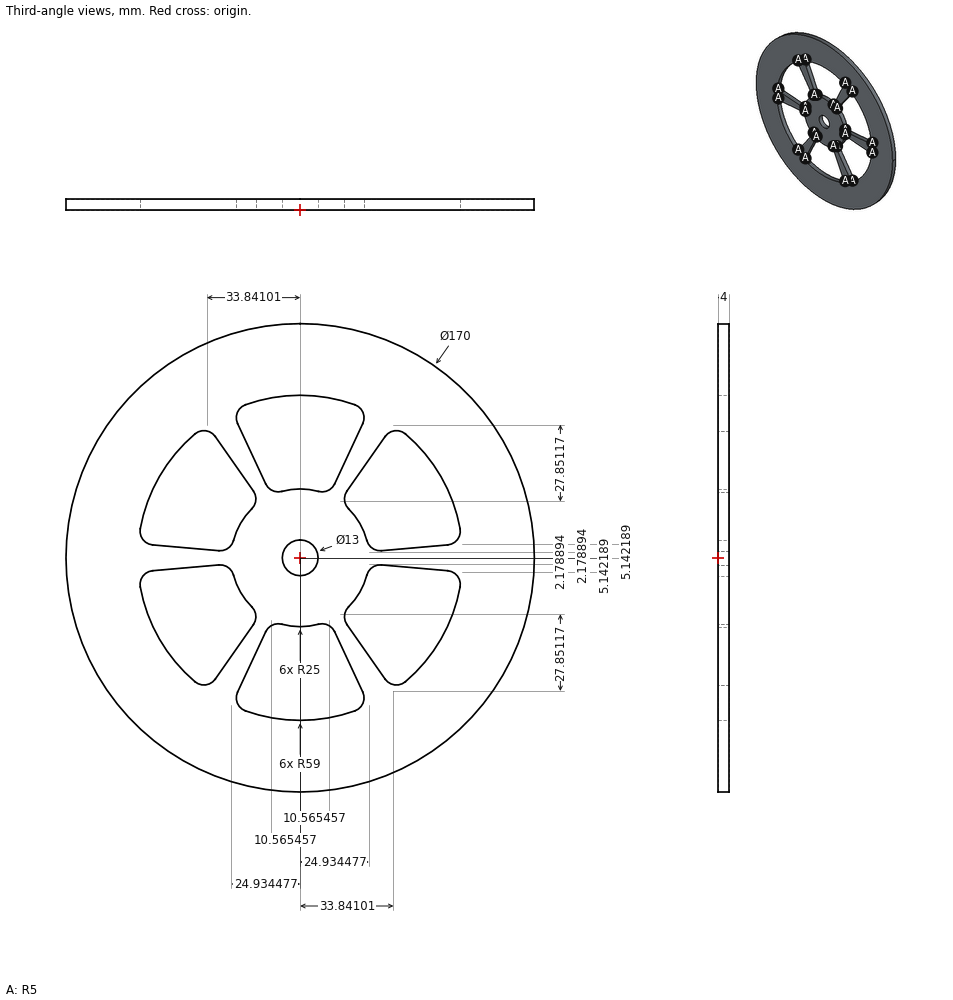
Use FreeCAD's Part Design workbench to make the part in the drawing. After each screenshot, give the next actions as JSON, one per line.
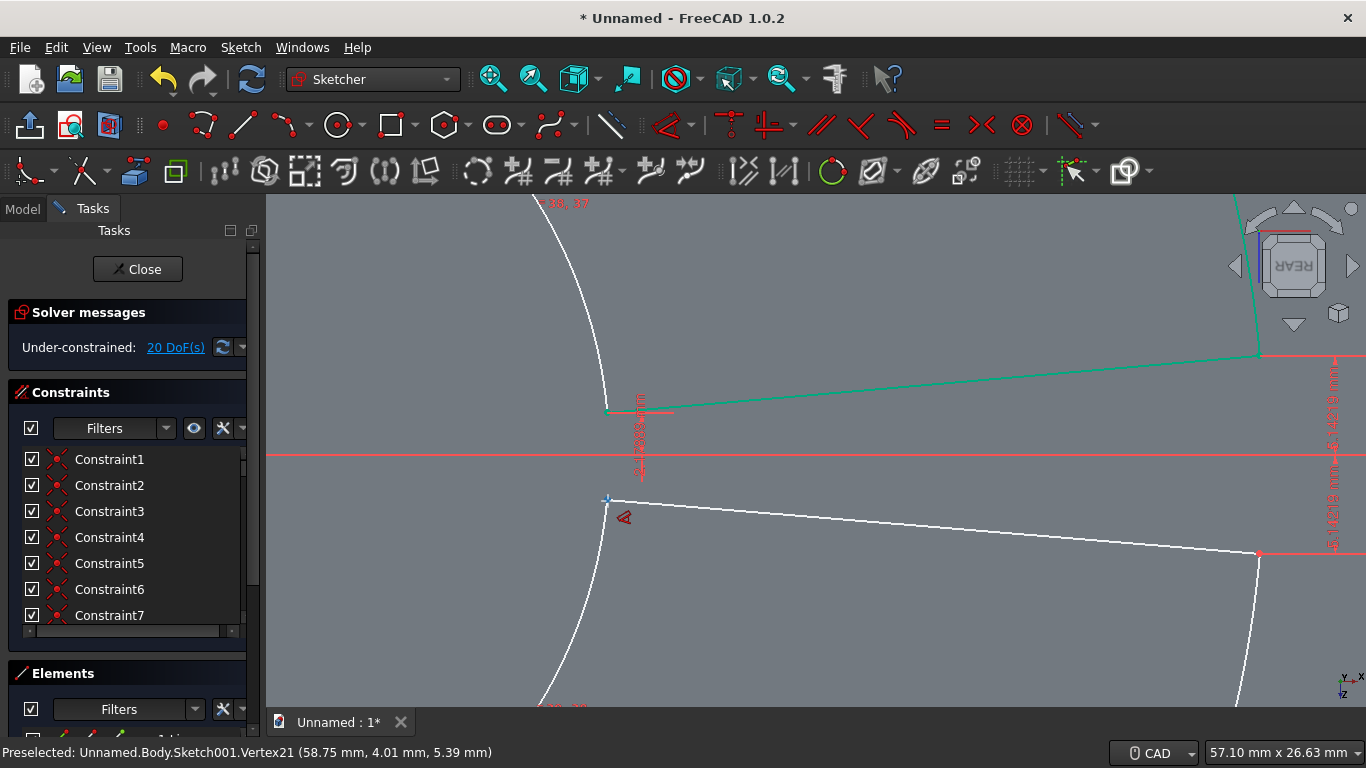
{"action": "left_click", "coordinate": [607, 500]}
{"action": "left_click", "coordinate": [641, 477]}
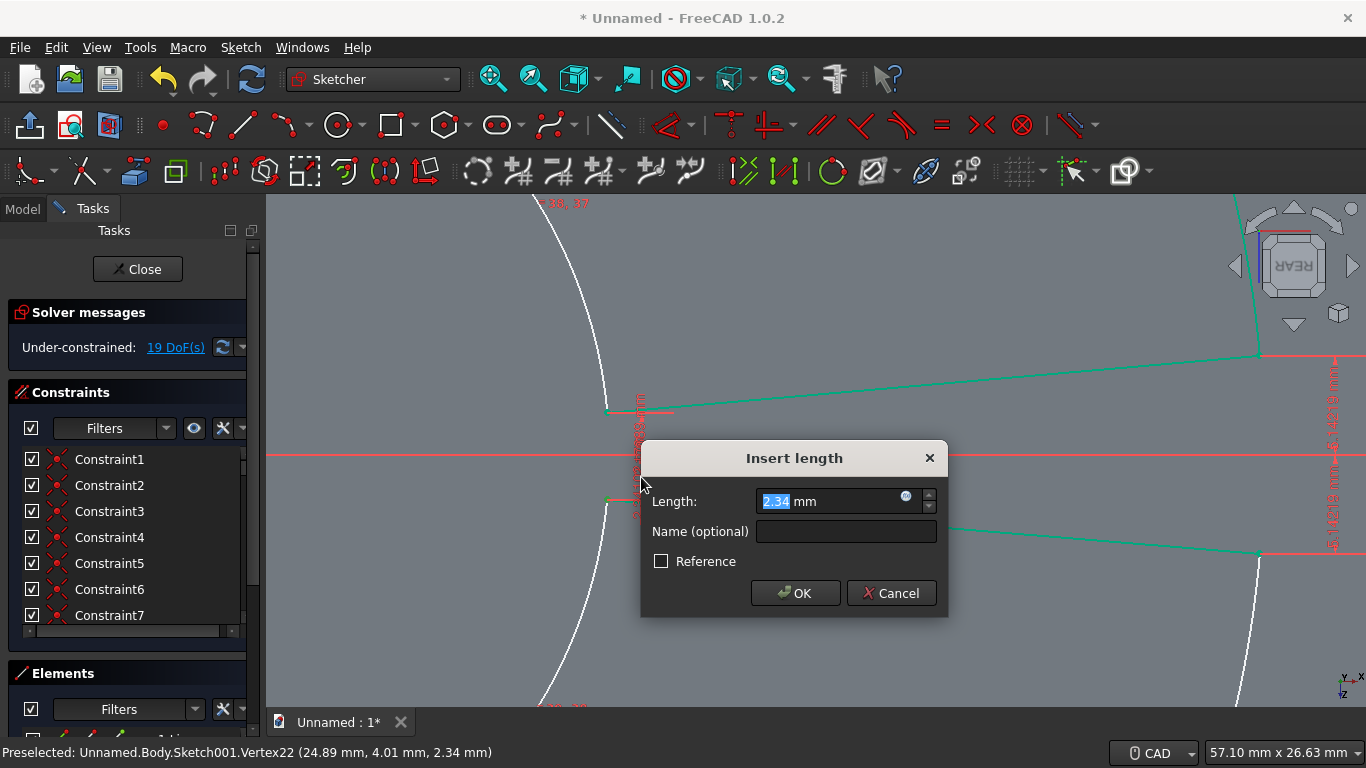
{"action": "type", "text": "2.178894"}
{"action": "key", "text": "Return"}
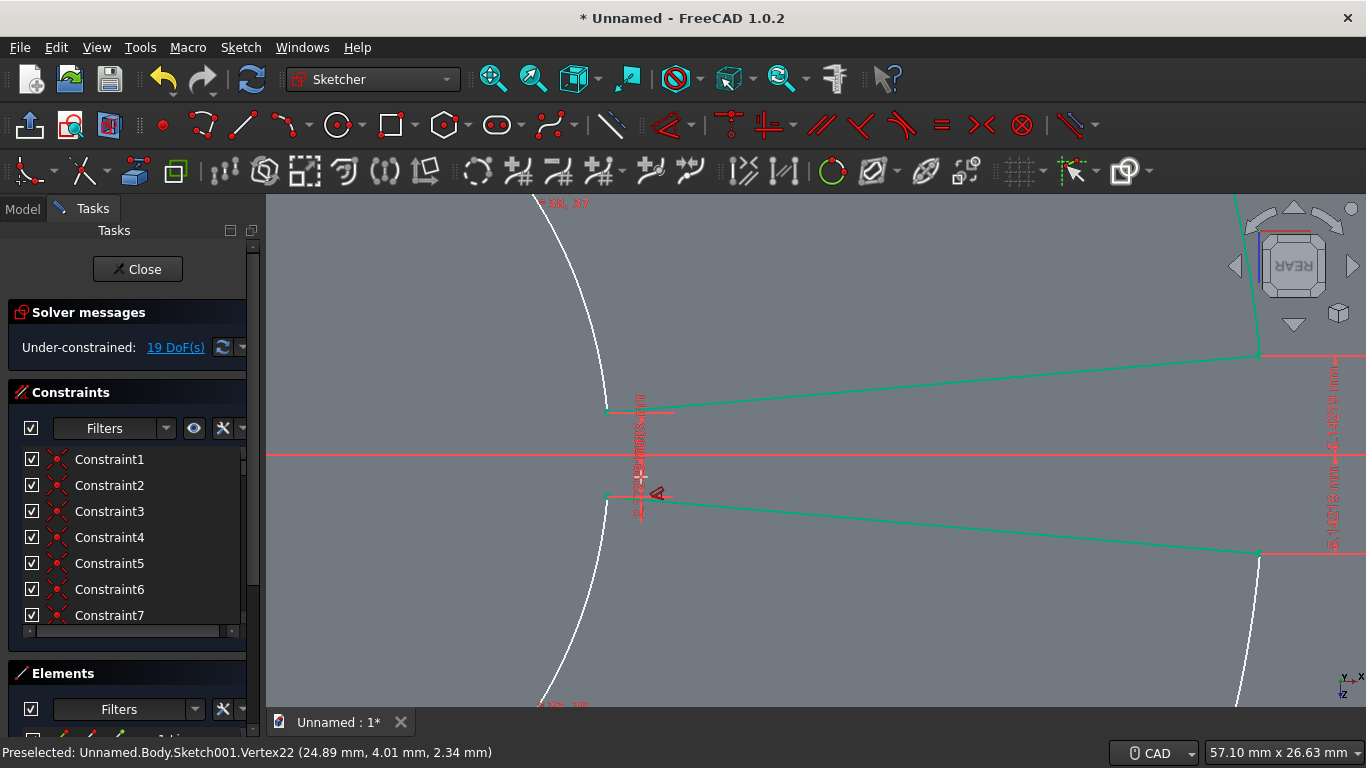
{"action": "scroll", "coordinate": [845, 450], "scroll_direction": "down", "scroll_amount": 10}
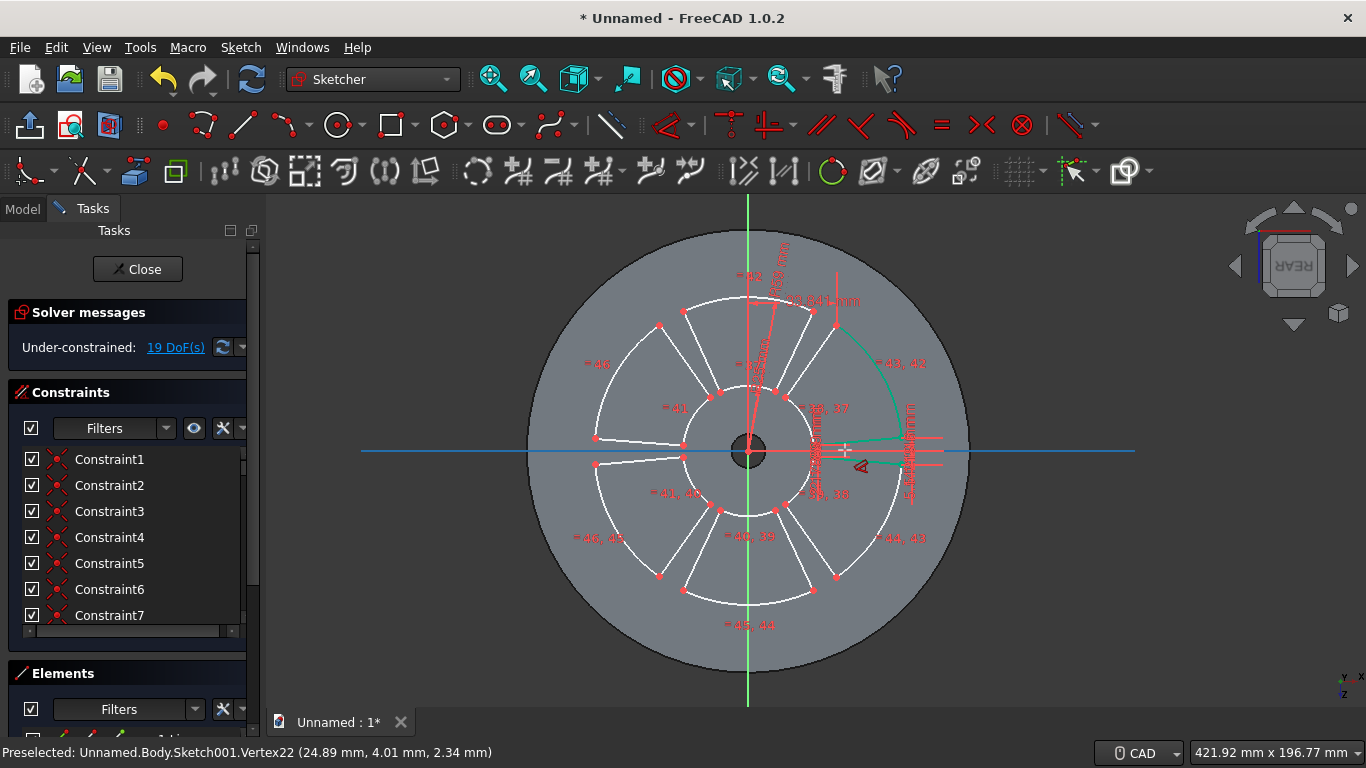
{"action": "left_click", "coordinate": [836, 577]}
{"action": "left_click", "coordinate": [813, 611]}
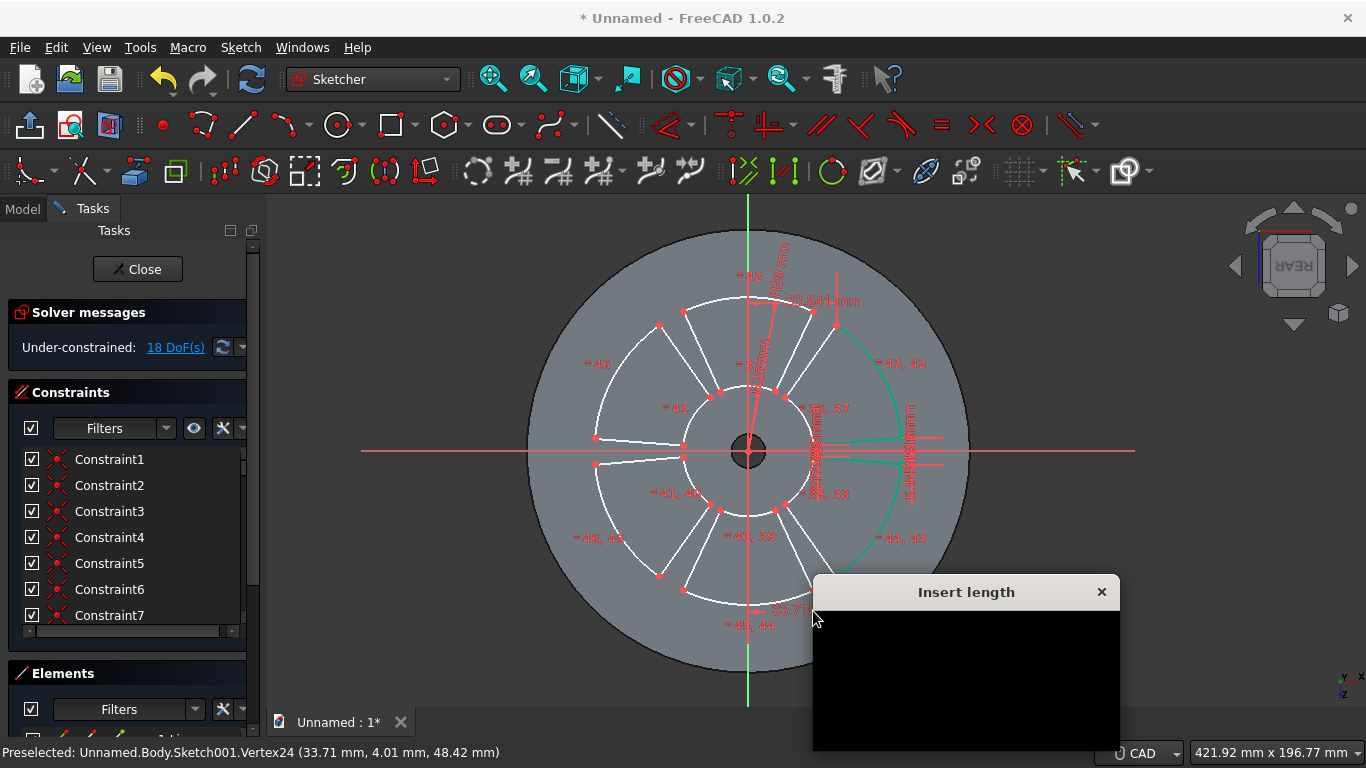
{"action": "type", "text": "33.84101"}
{"action": "key", "text": "Return"}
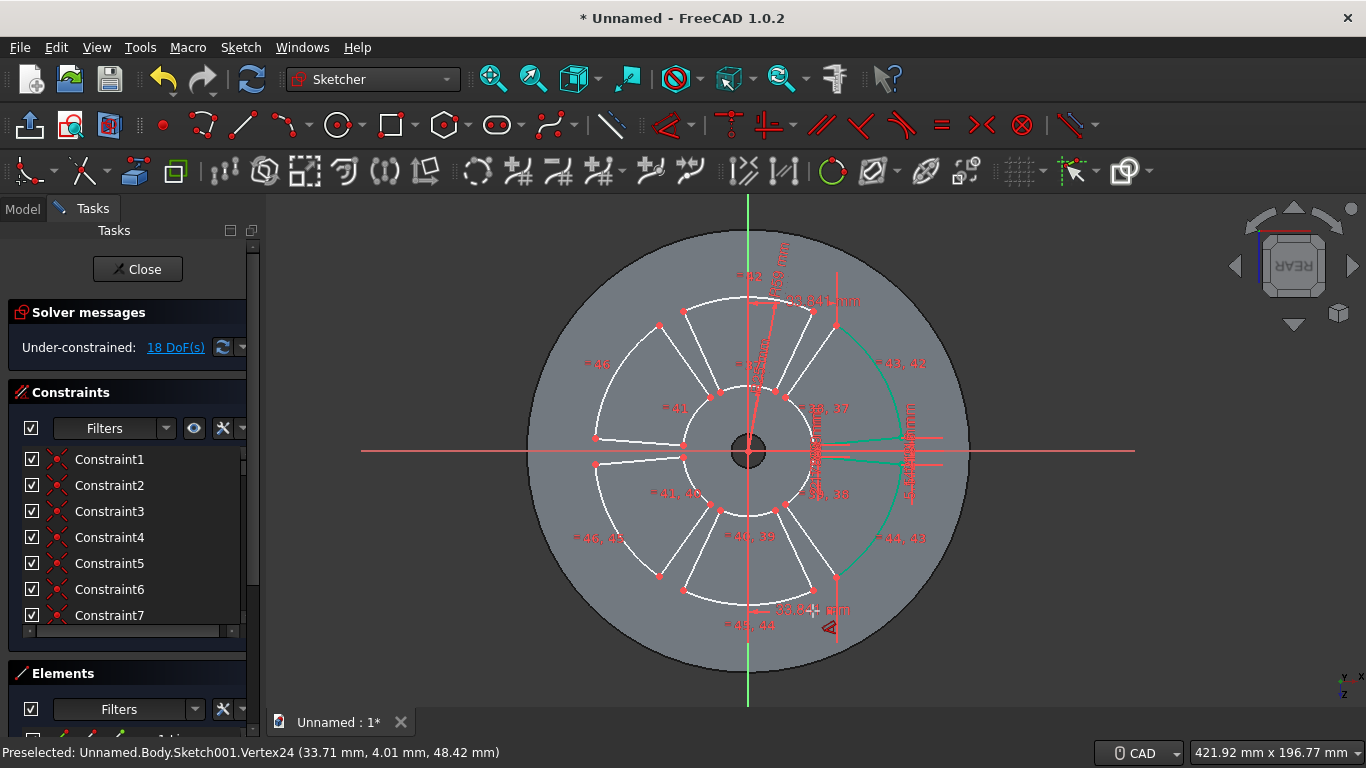
{"action": "left_click", "coordinate": [660, 577]}
{"action": "left_click", "coordinate": [684, 611]}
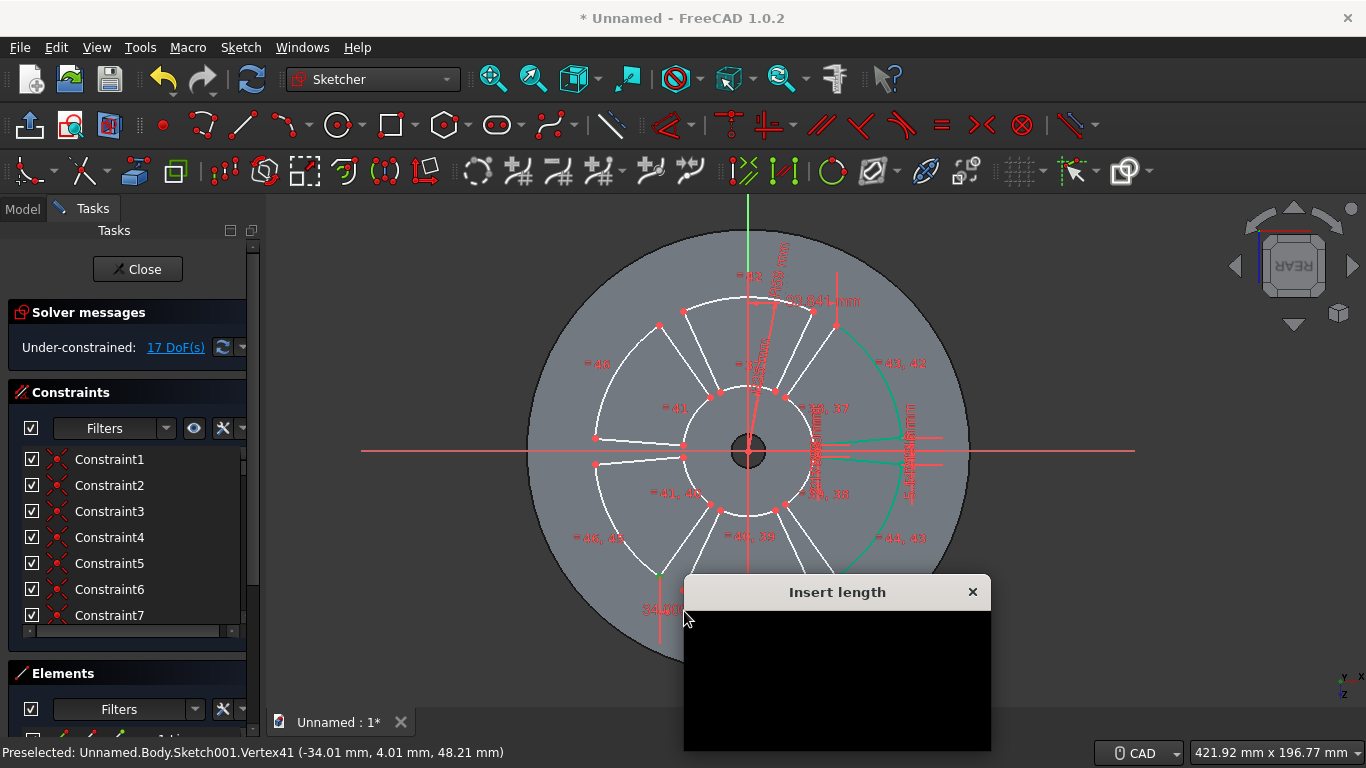
{"action": "type", "text": "33.84101"}
{"action": "key", "text": "Return"}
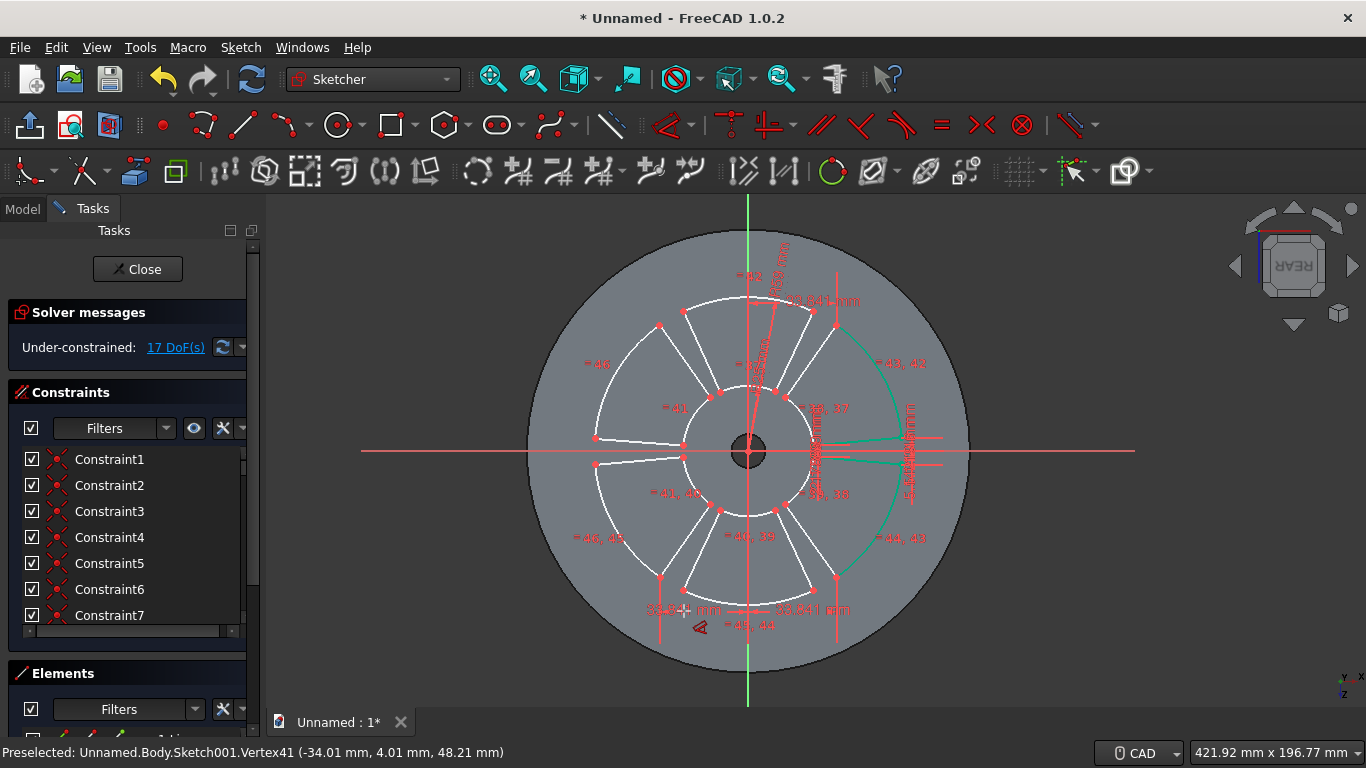
{"action": "scroll", "coordinate": [683, 457], "scroll_direction": "up", "scroll_amount": 10}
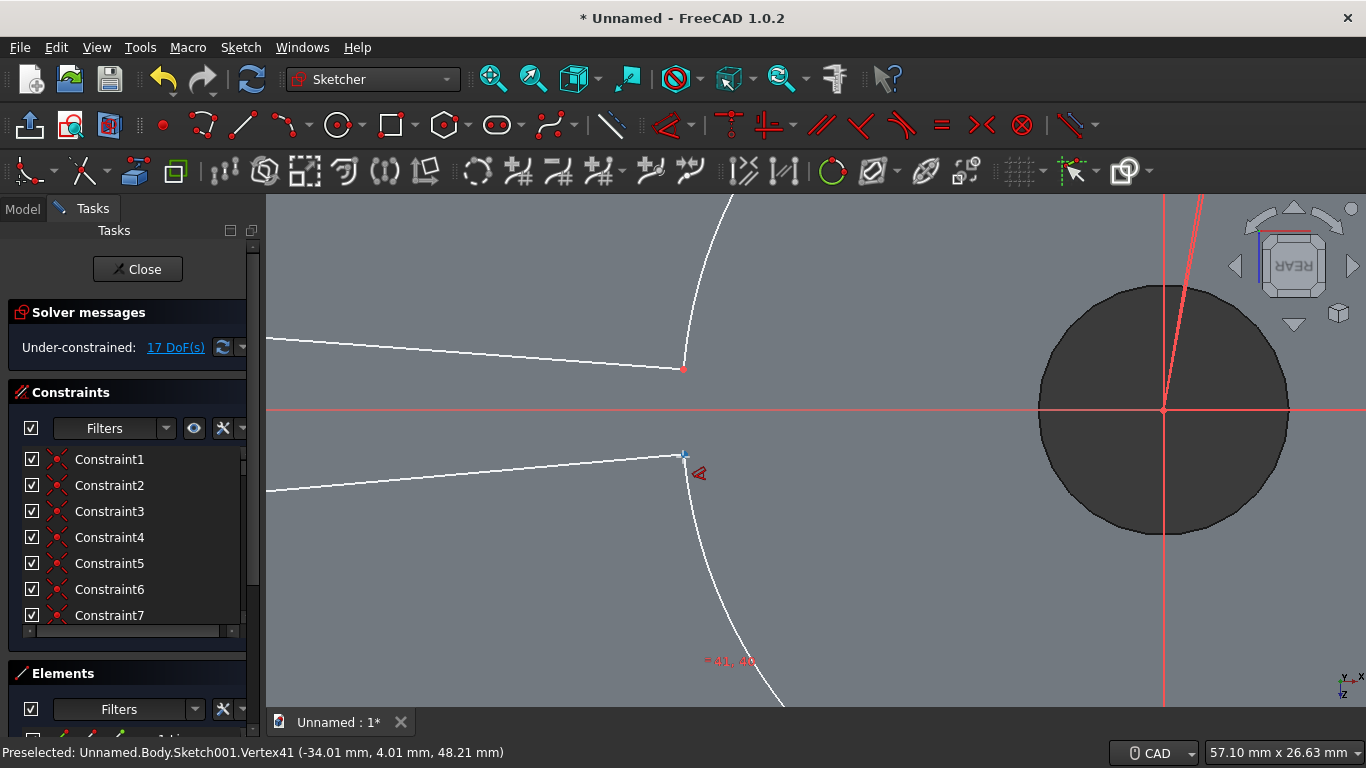
{"action": "left_click", "coordinate": [684, 454]}
{"action": "left_click", "coordinate": [650, 432]}